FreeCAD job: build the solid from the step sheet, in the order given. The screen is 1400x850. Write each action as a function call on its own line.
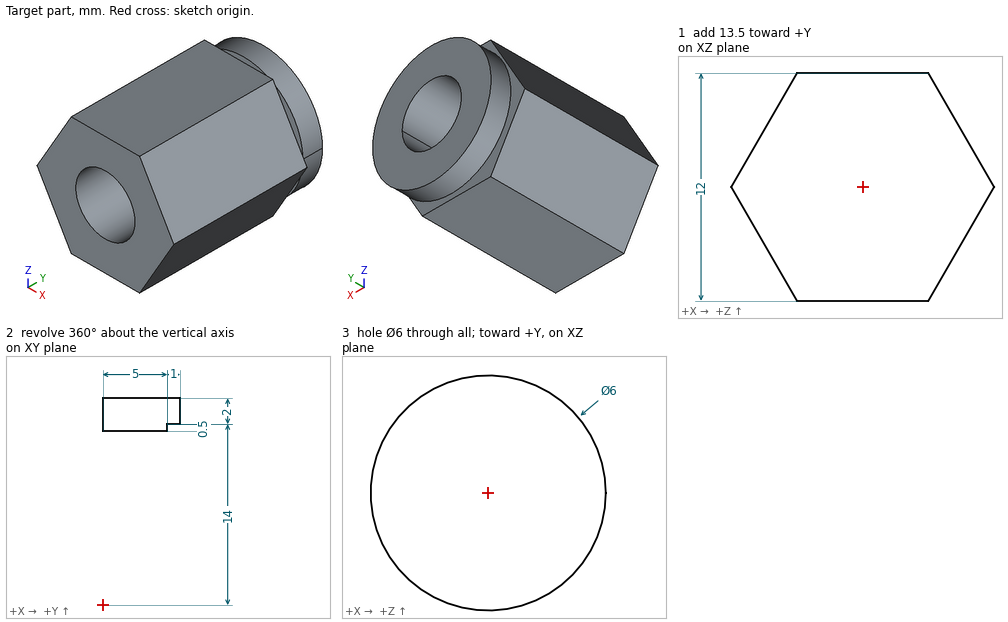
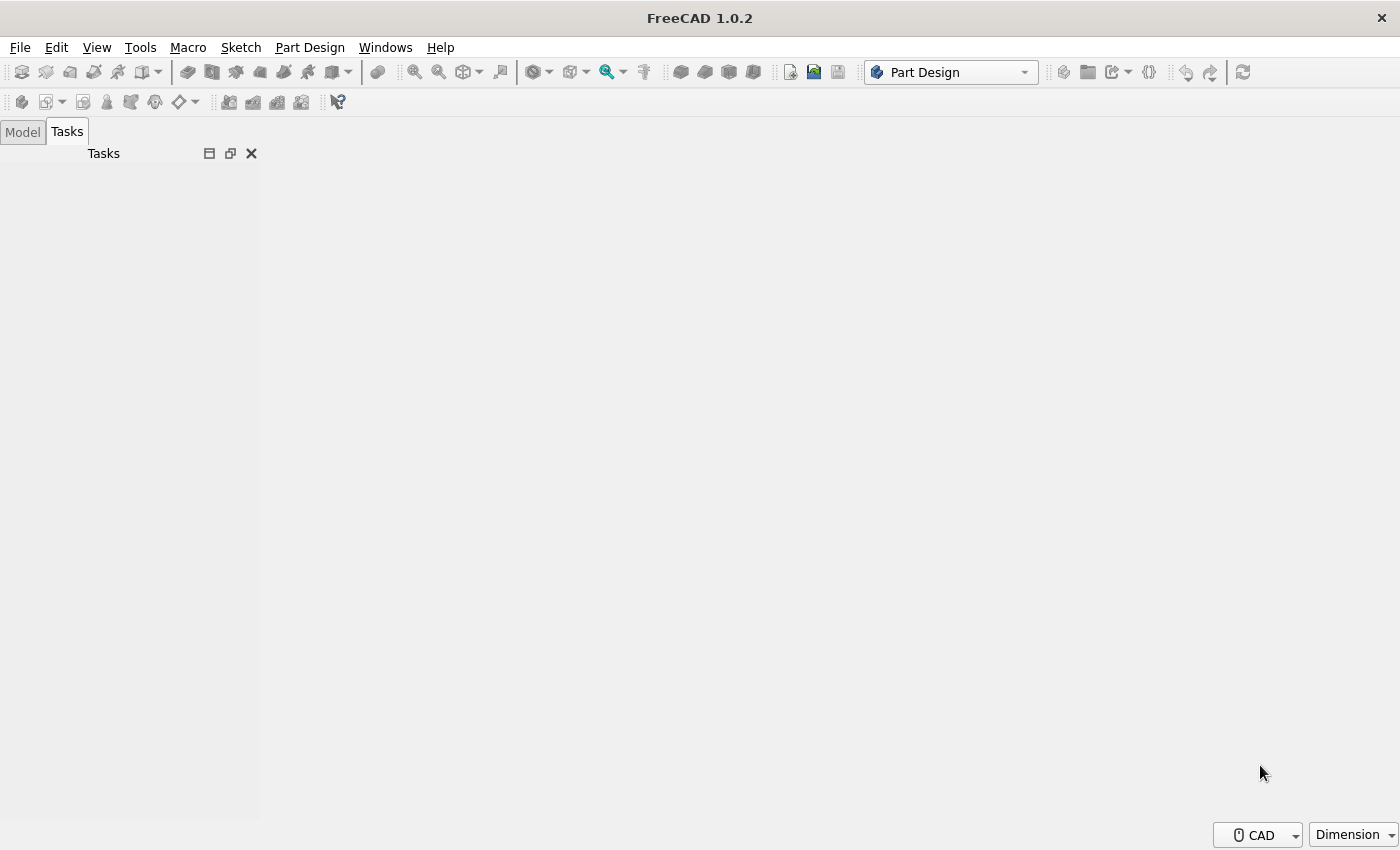
click(790, 72)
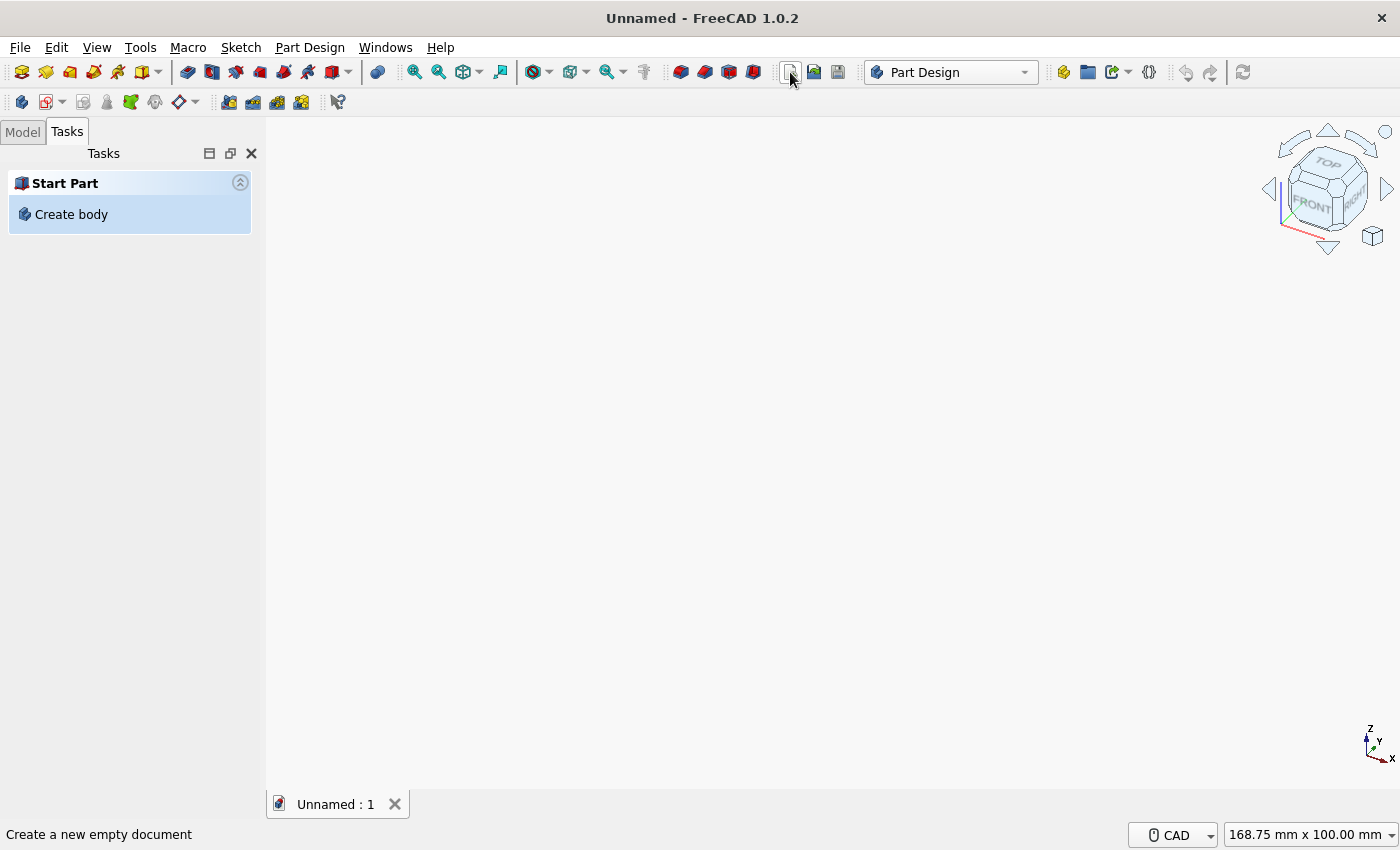
click(46, 102)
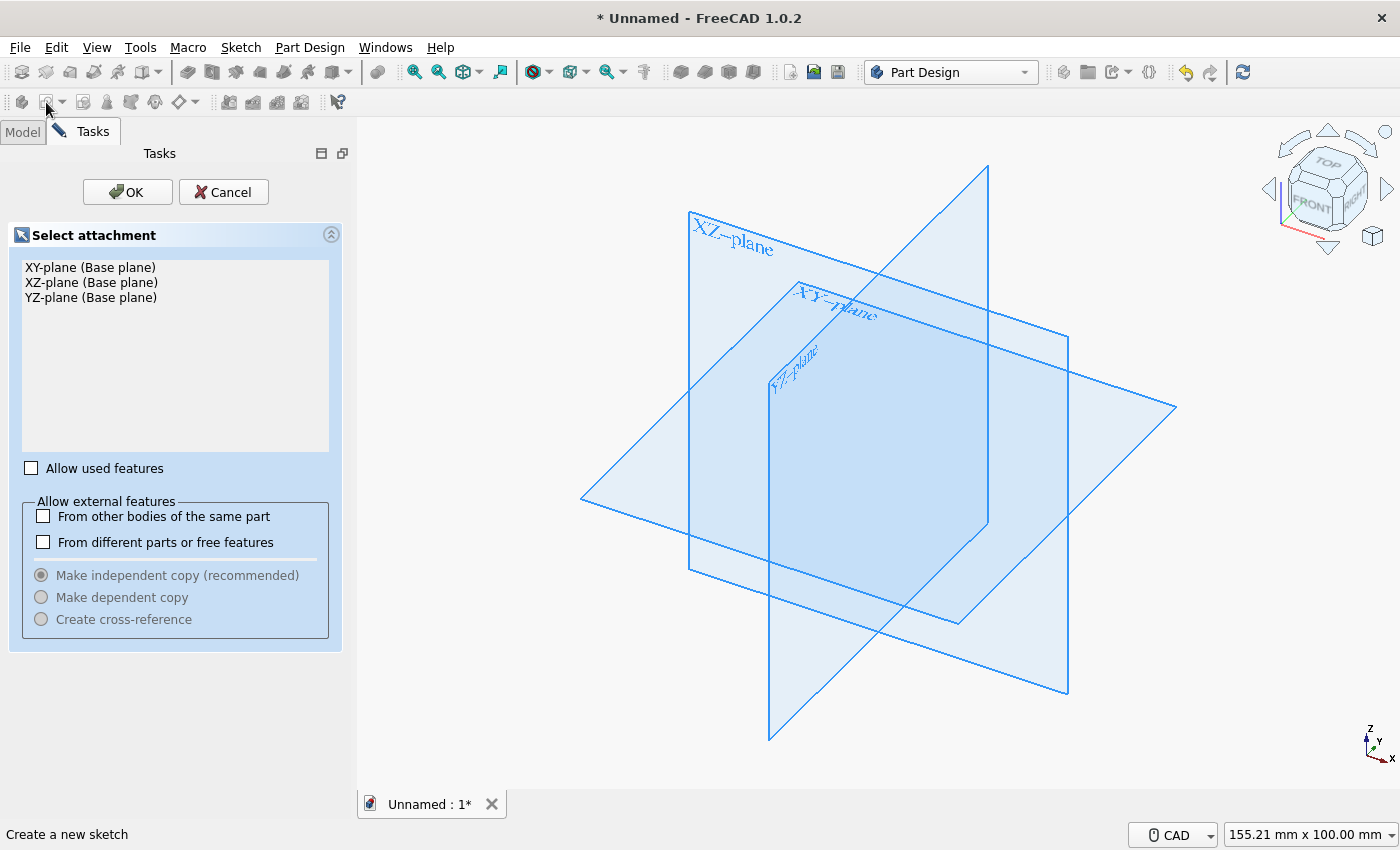
click(82, 282)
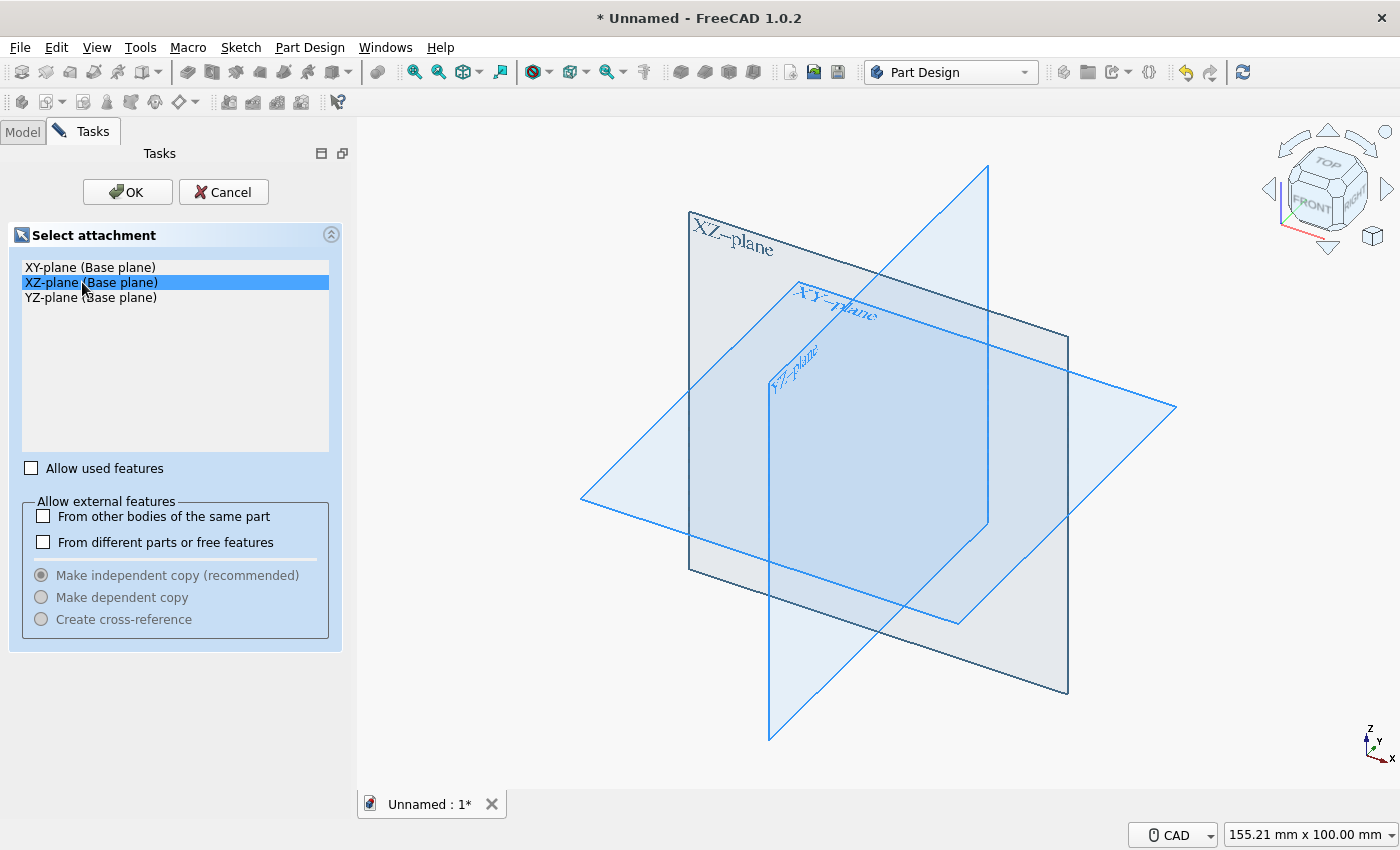
click(128, 192)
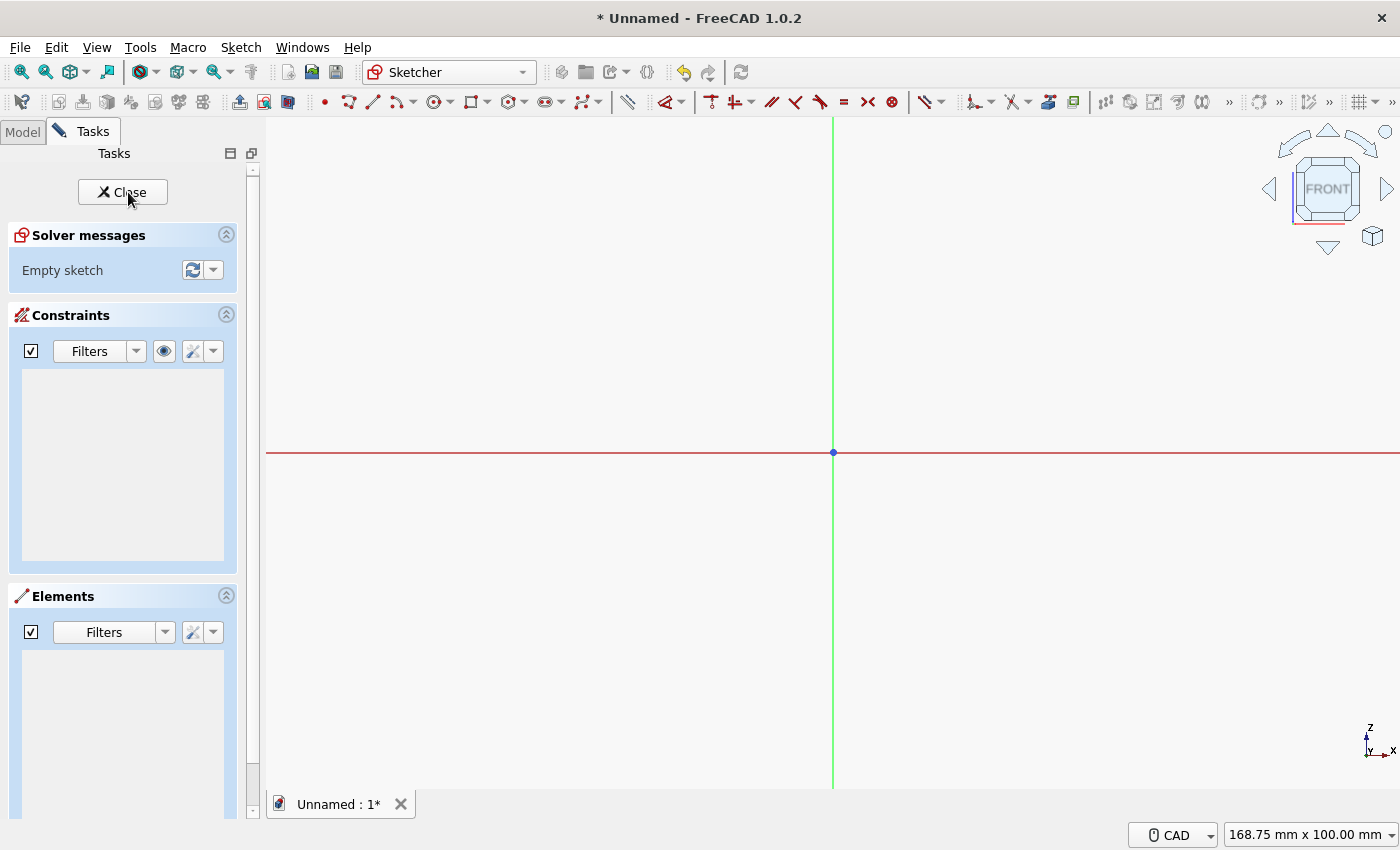
scroll(850, 453, up, 8)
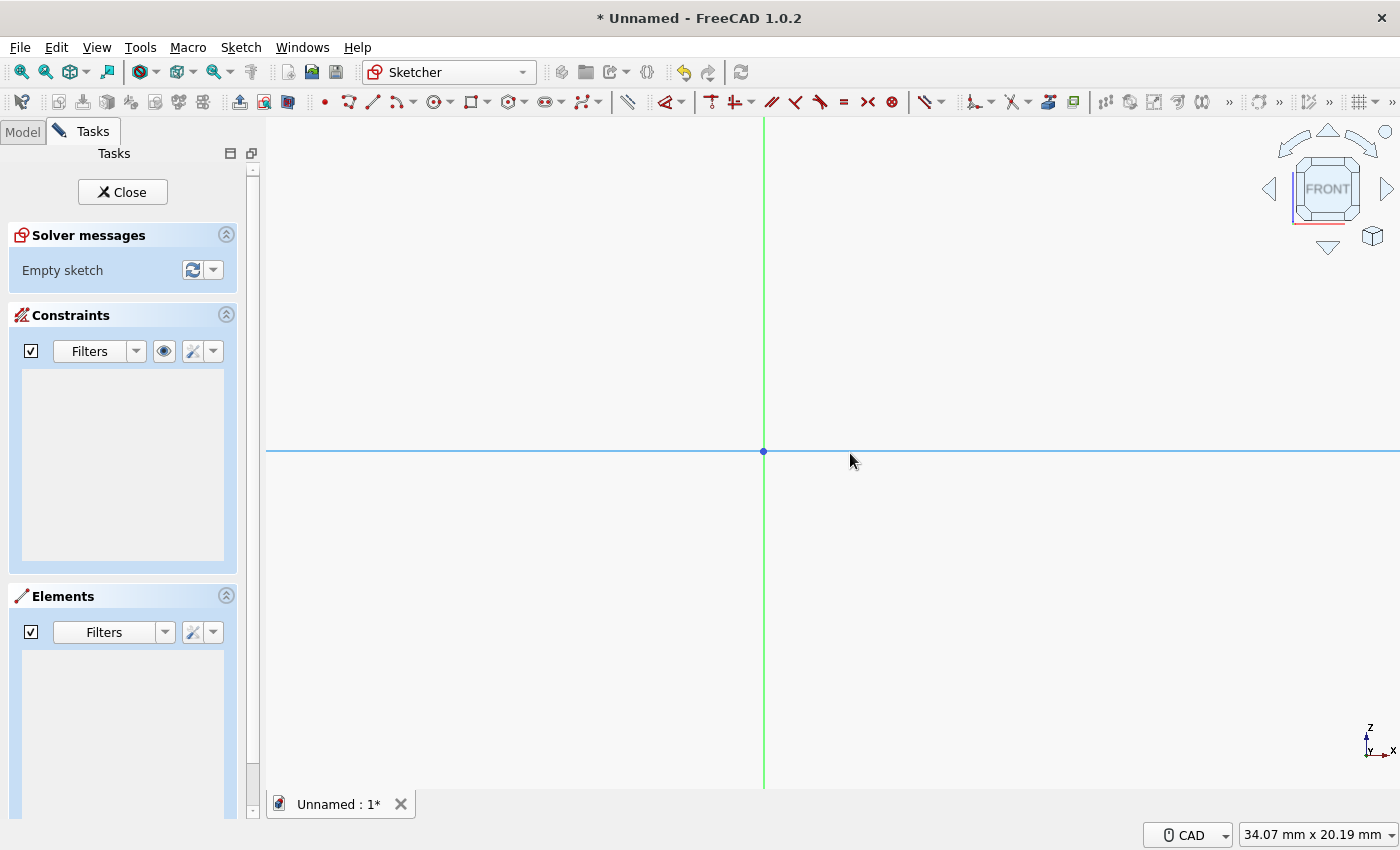
click(508, 102)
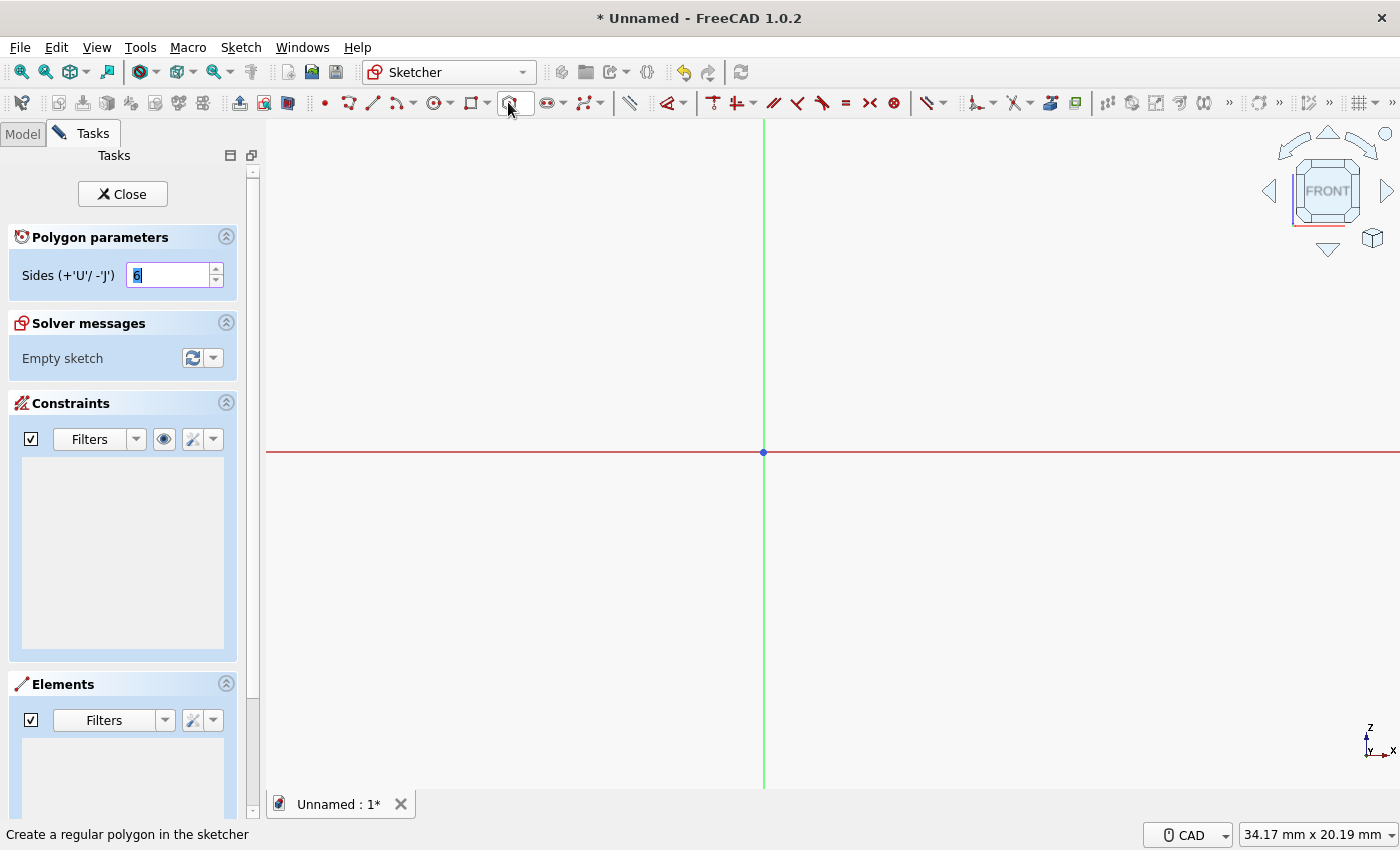
click(764, 452)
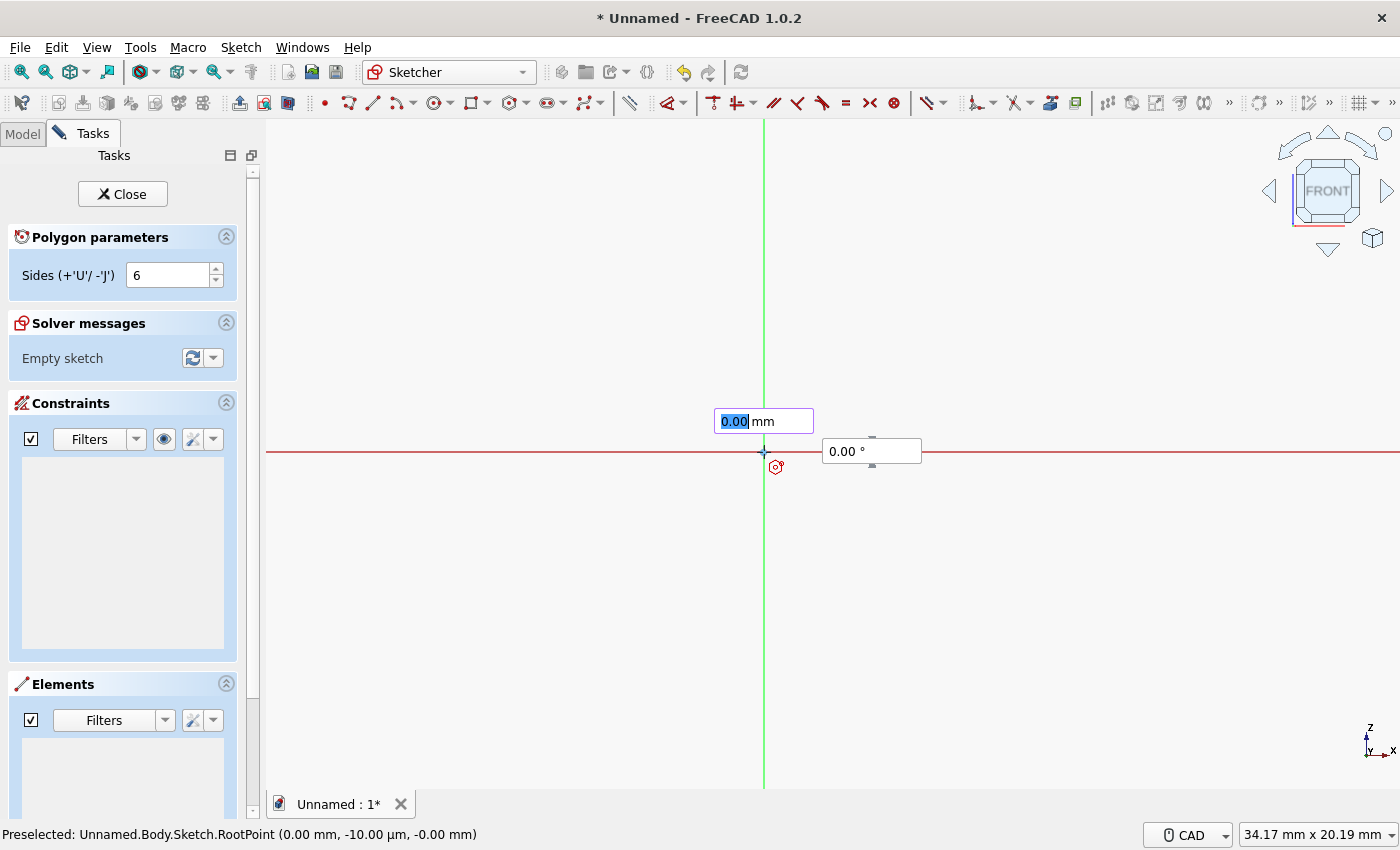
click(534, 452)
right_click(534, 452)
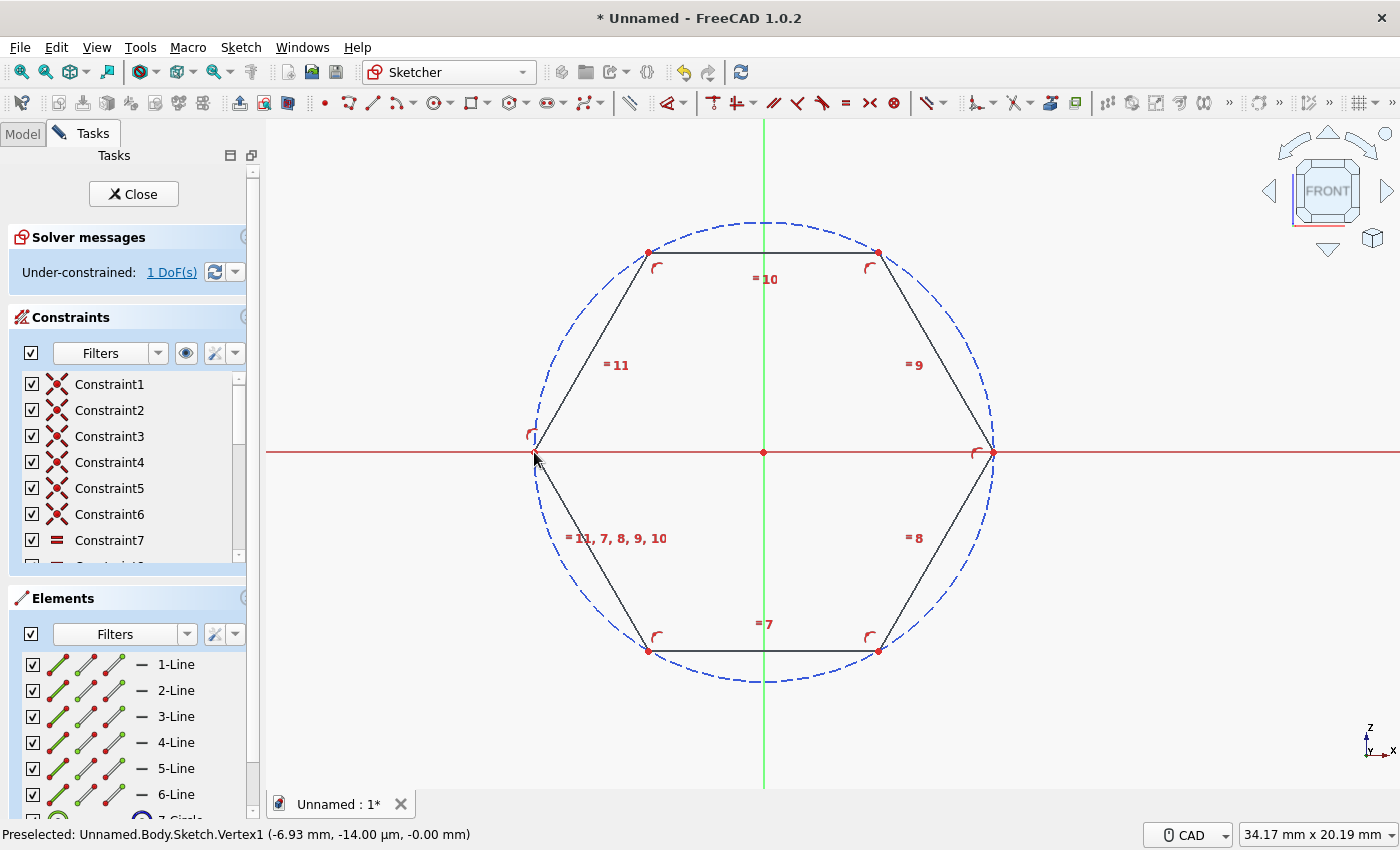
click(668, 104)